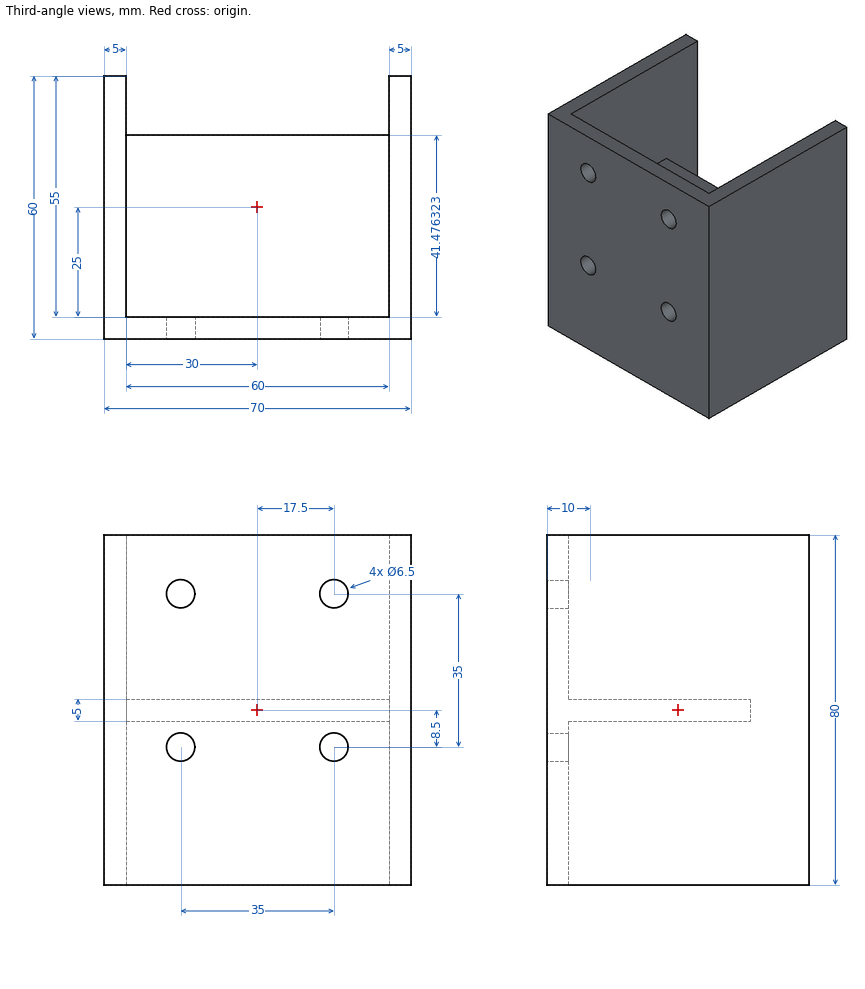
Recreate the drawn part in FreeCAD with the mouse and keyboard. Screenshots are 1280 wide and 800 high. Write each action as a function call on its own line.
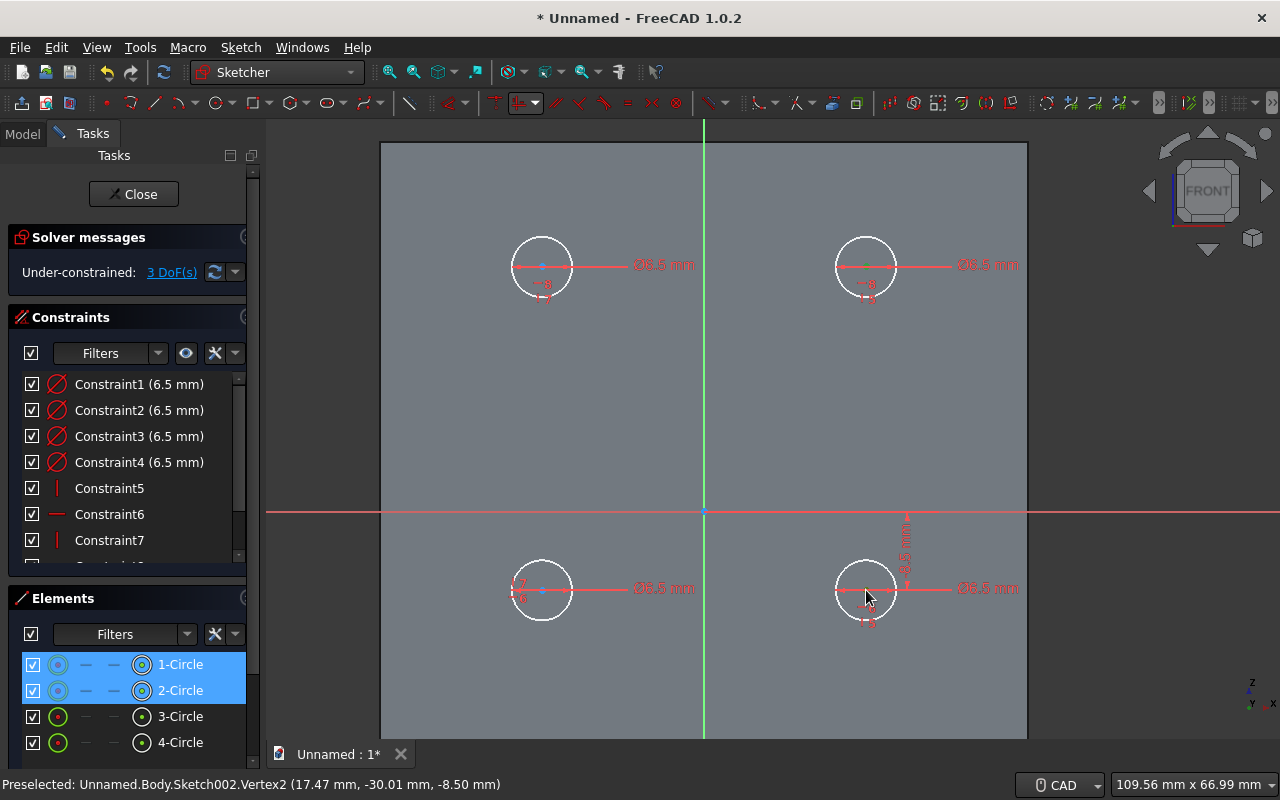
key(i)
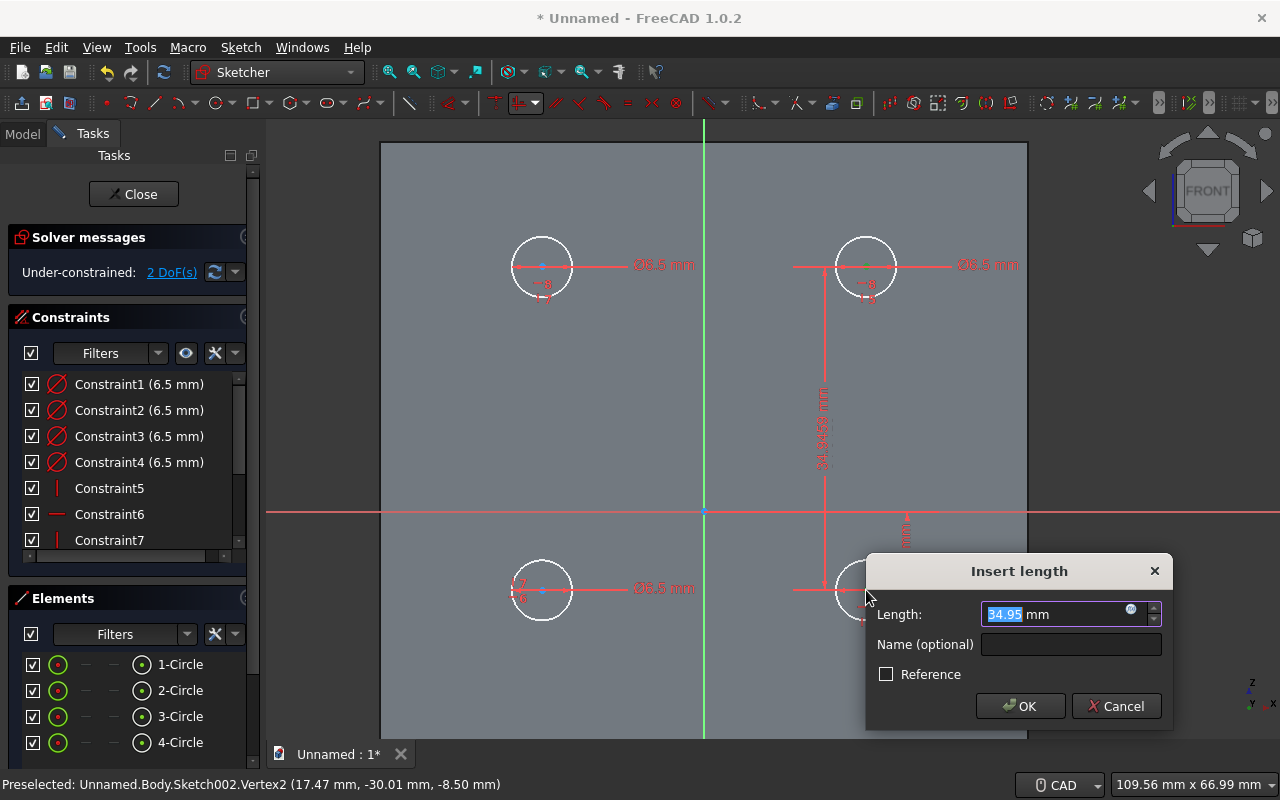
text(35)
key(Return)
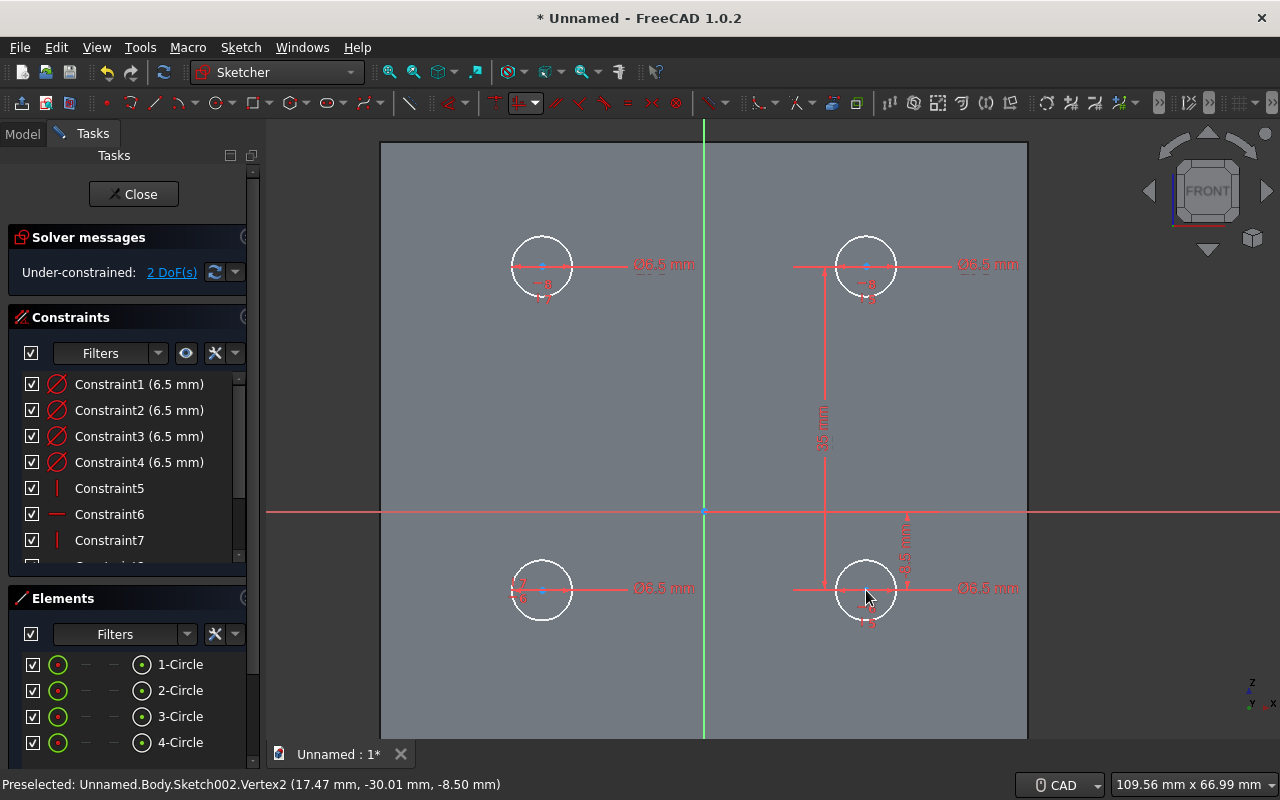
click(866, 590)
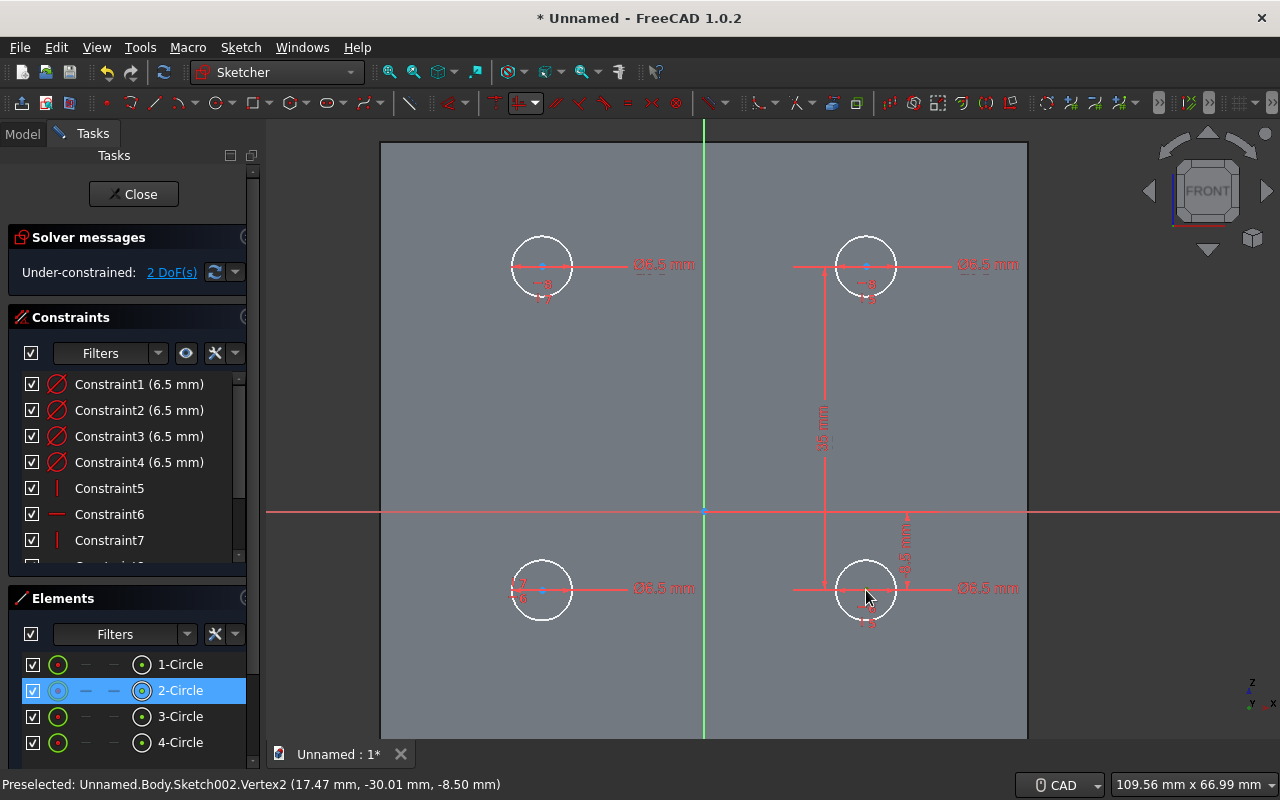
click(542, 590)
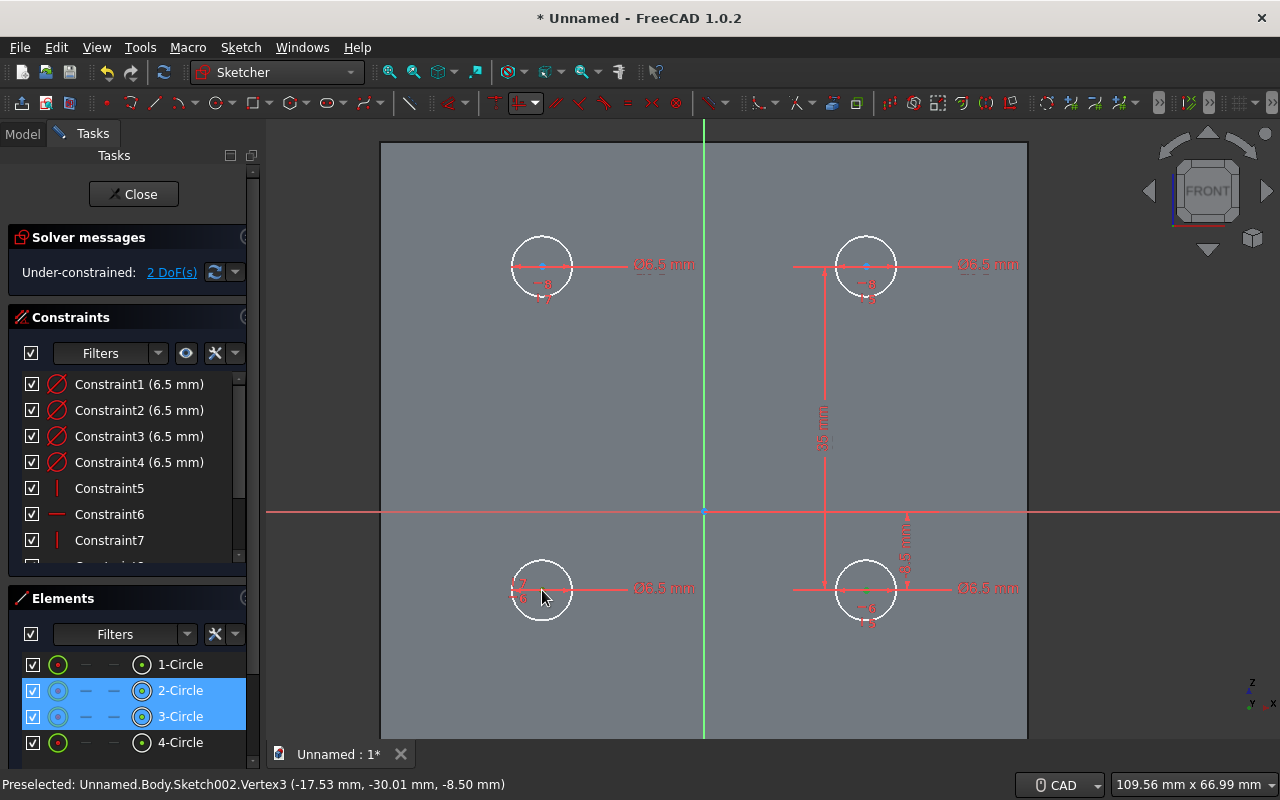
key(l)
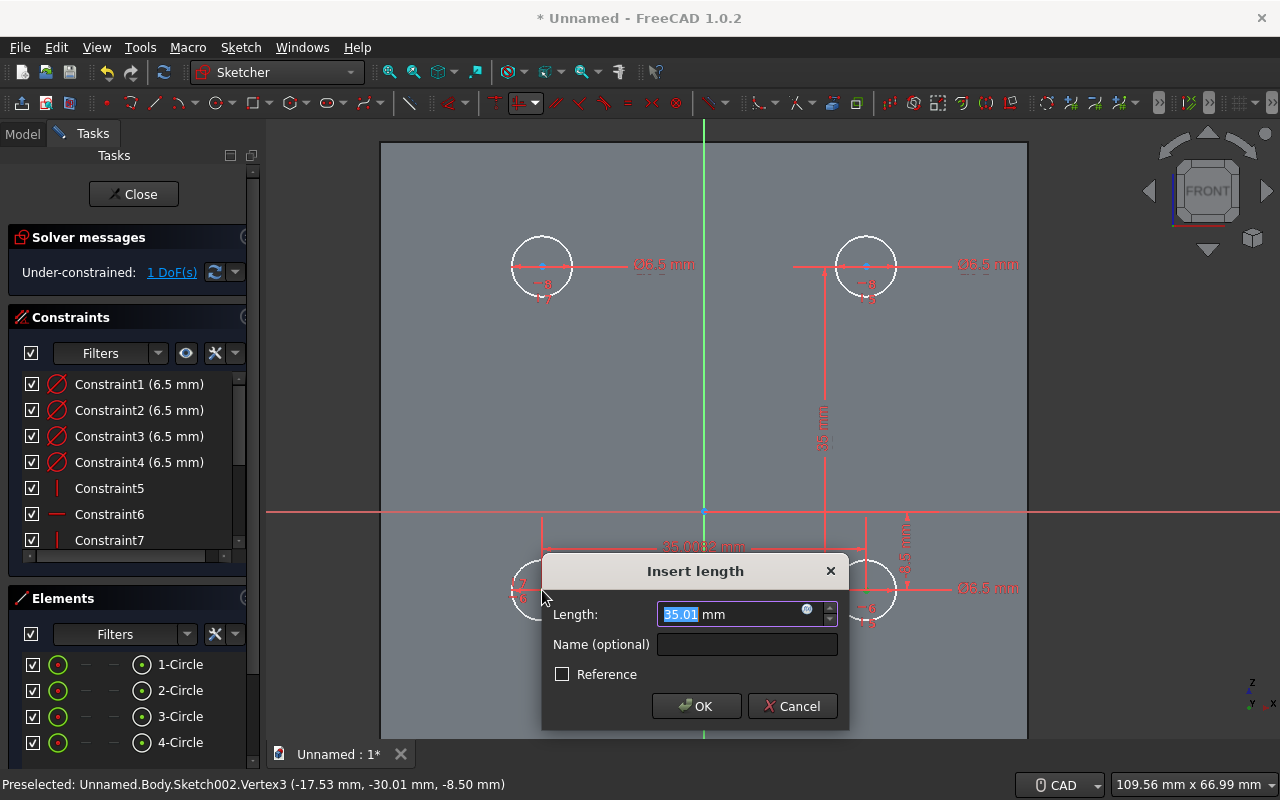
text(35)
key(Return)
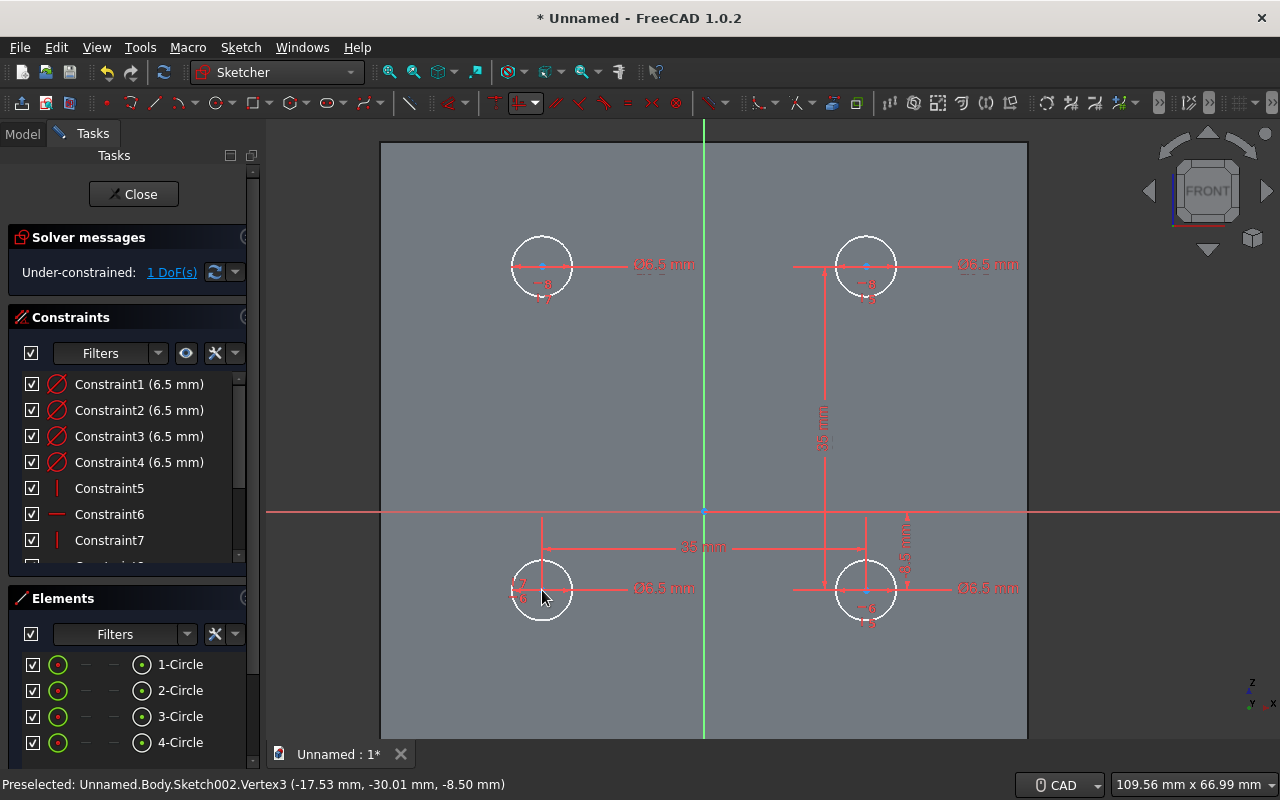
click(866, 266)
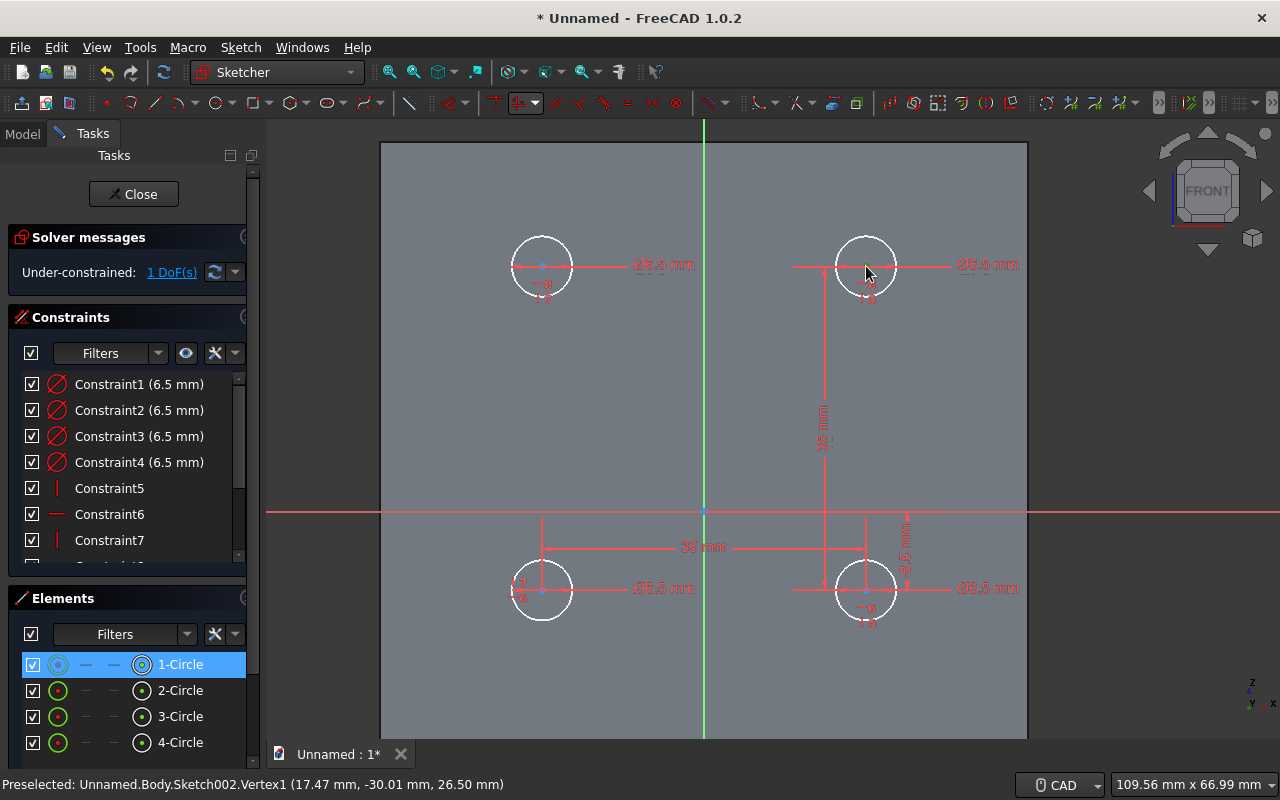
key(l)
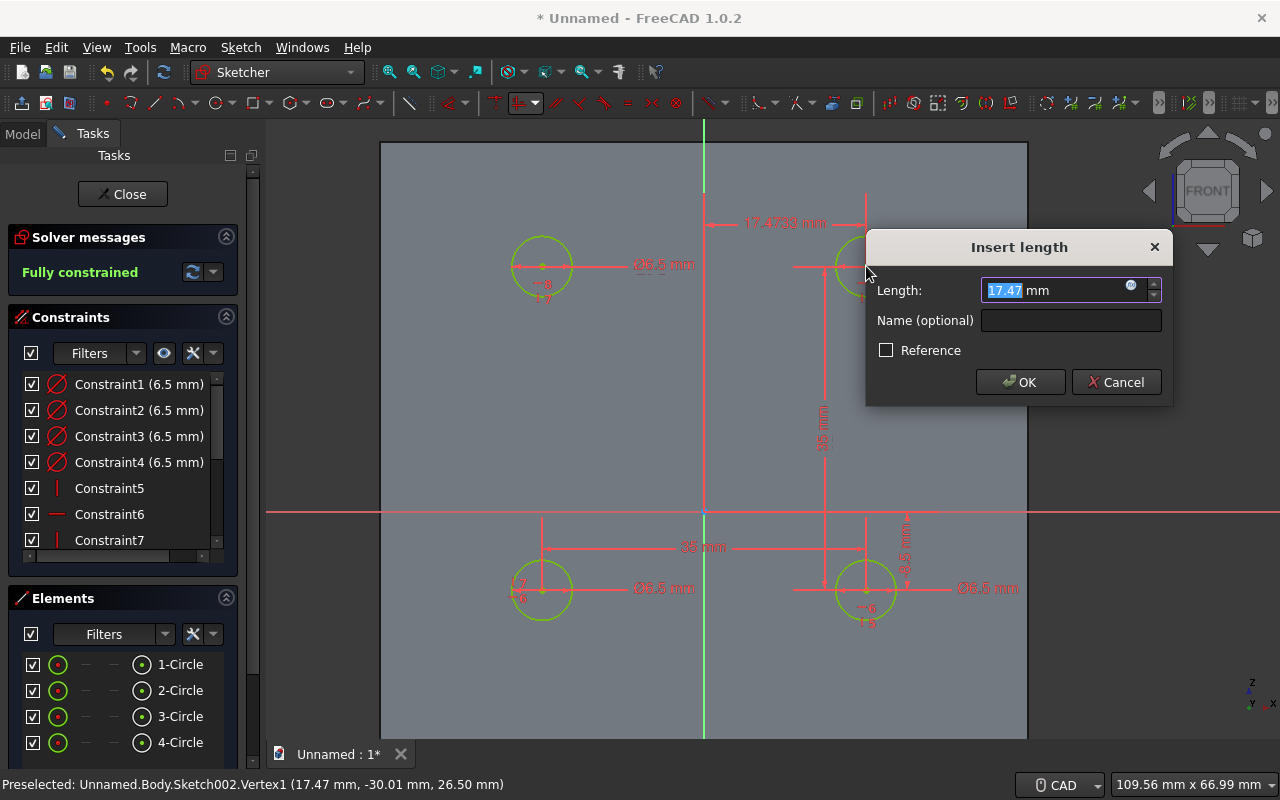
text(17.5)
key(Return)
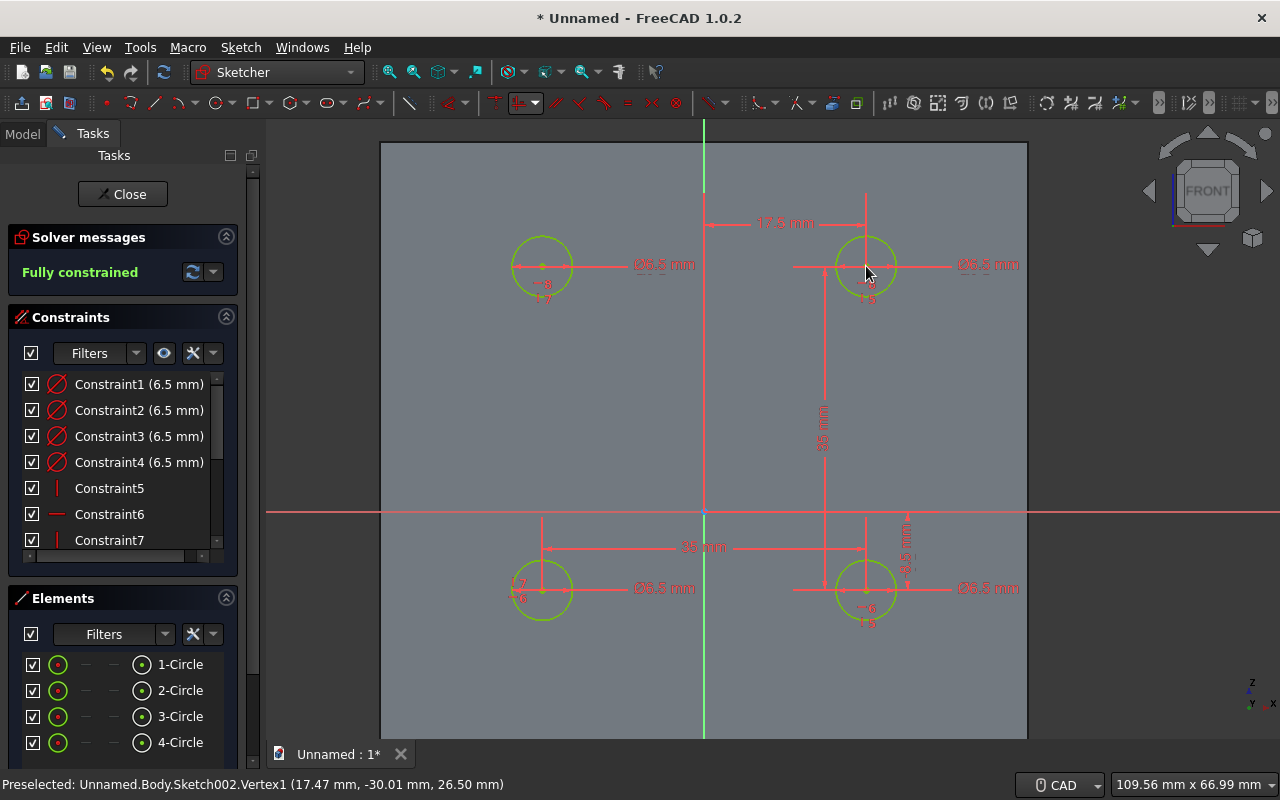
click(123, 194)